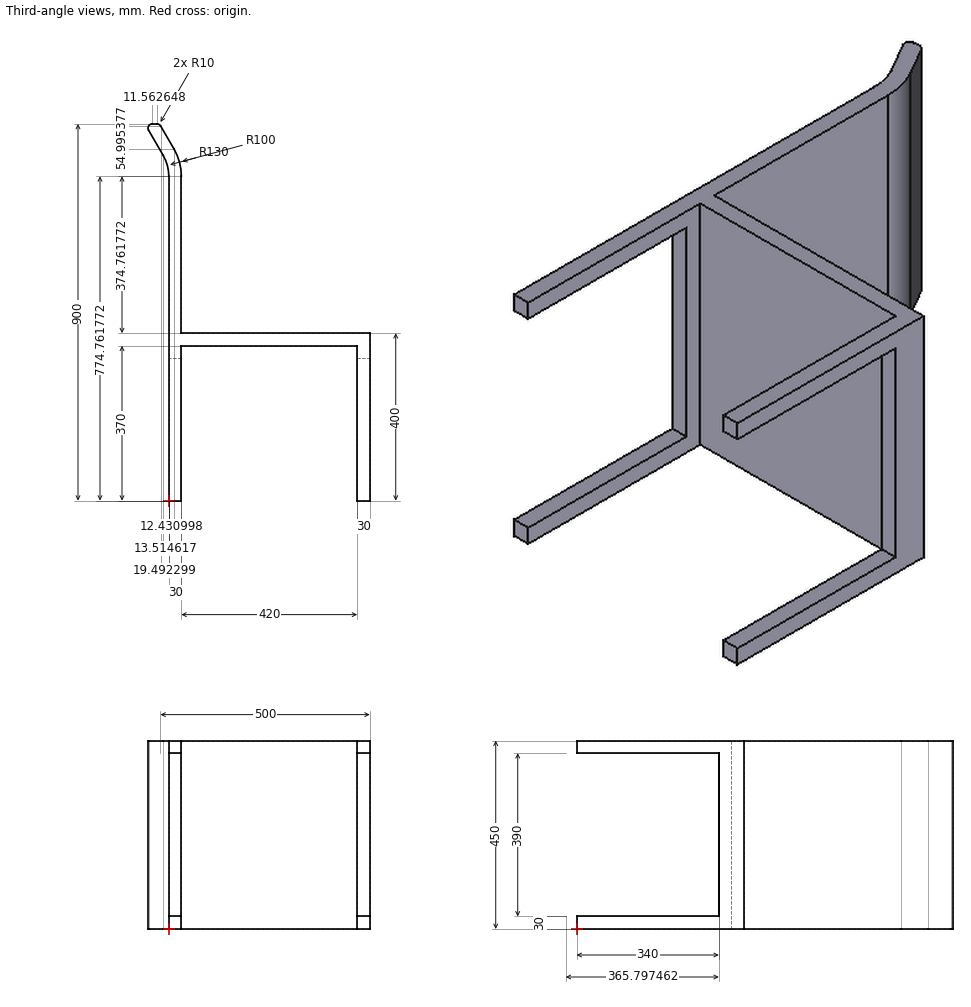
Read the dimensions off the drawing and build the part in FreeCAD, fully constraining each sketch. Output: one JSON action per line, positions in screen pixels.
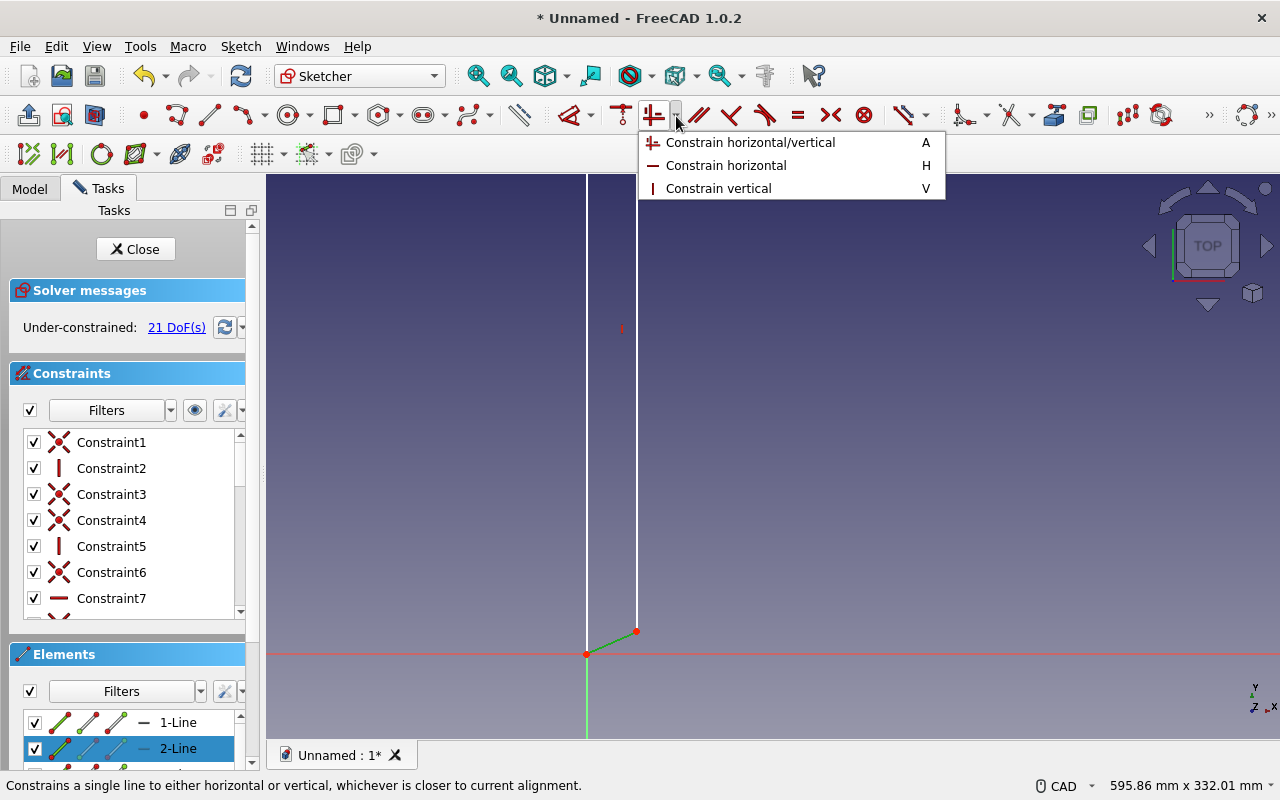
{"action": "left_click", "coordinate": [792, 166]}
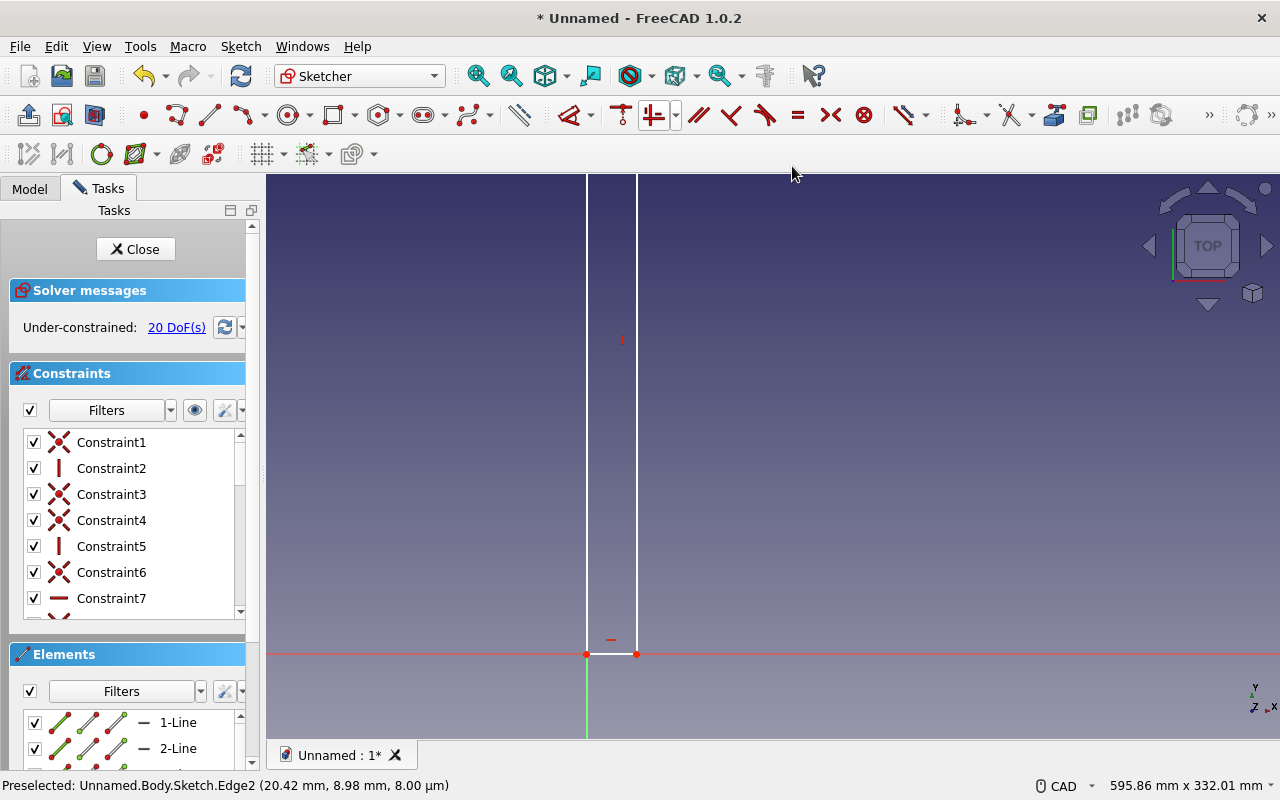
{"action": "scroll", "coordinate": [623, 642], "scroll_direction": "down", "scroll_amount": 7}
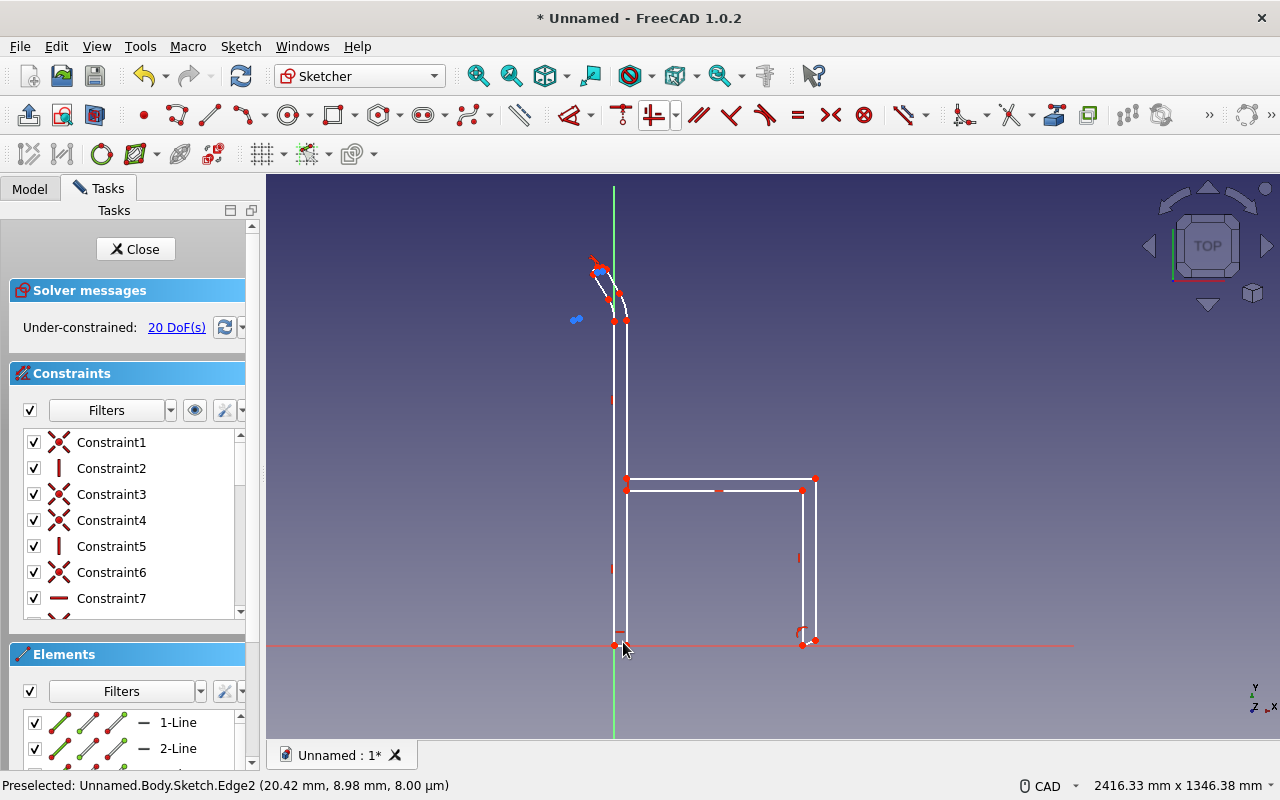
{"action": "scroll", "coordinate": [812, 642], "scroll_direction": "up", "scroll_amount": 7}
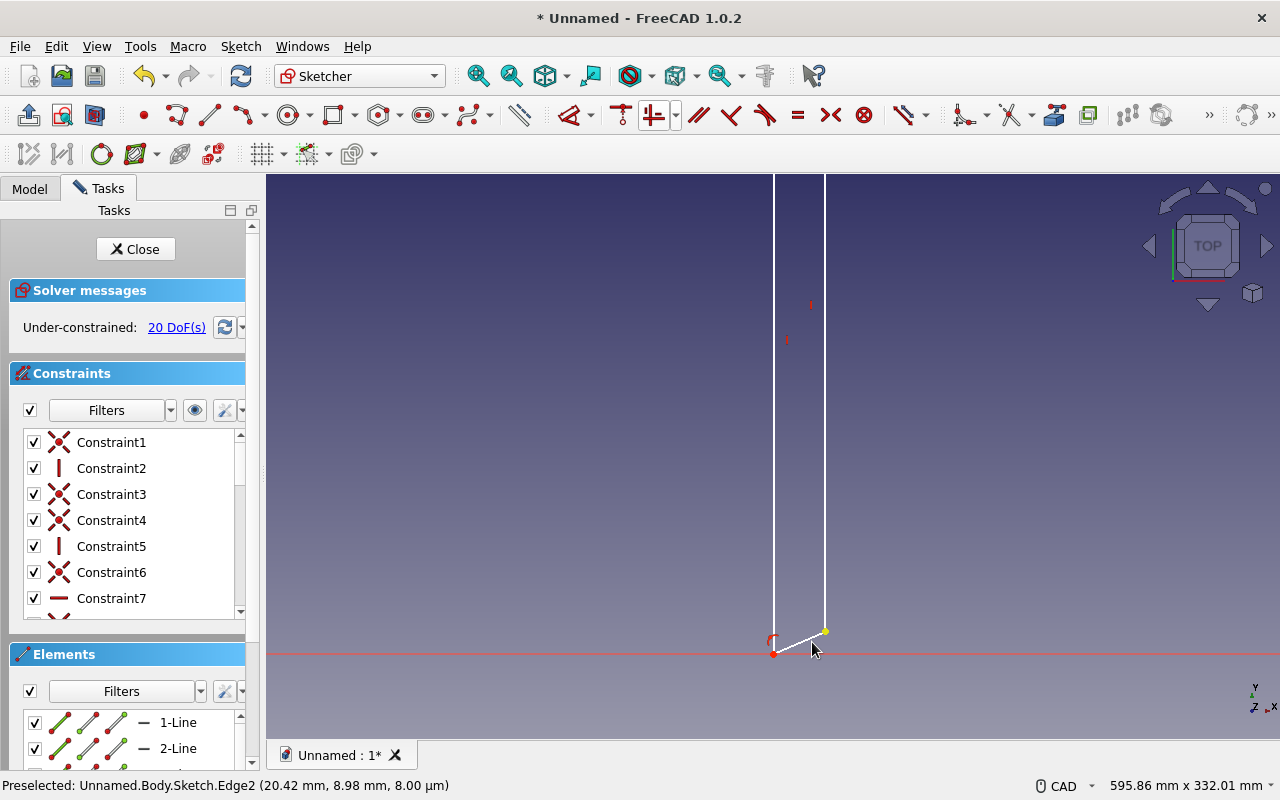
{"action": "left_click", "coordinate": [810, 639]}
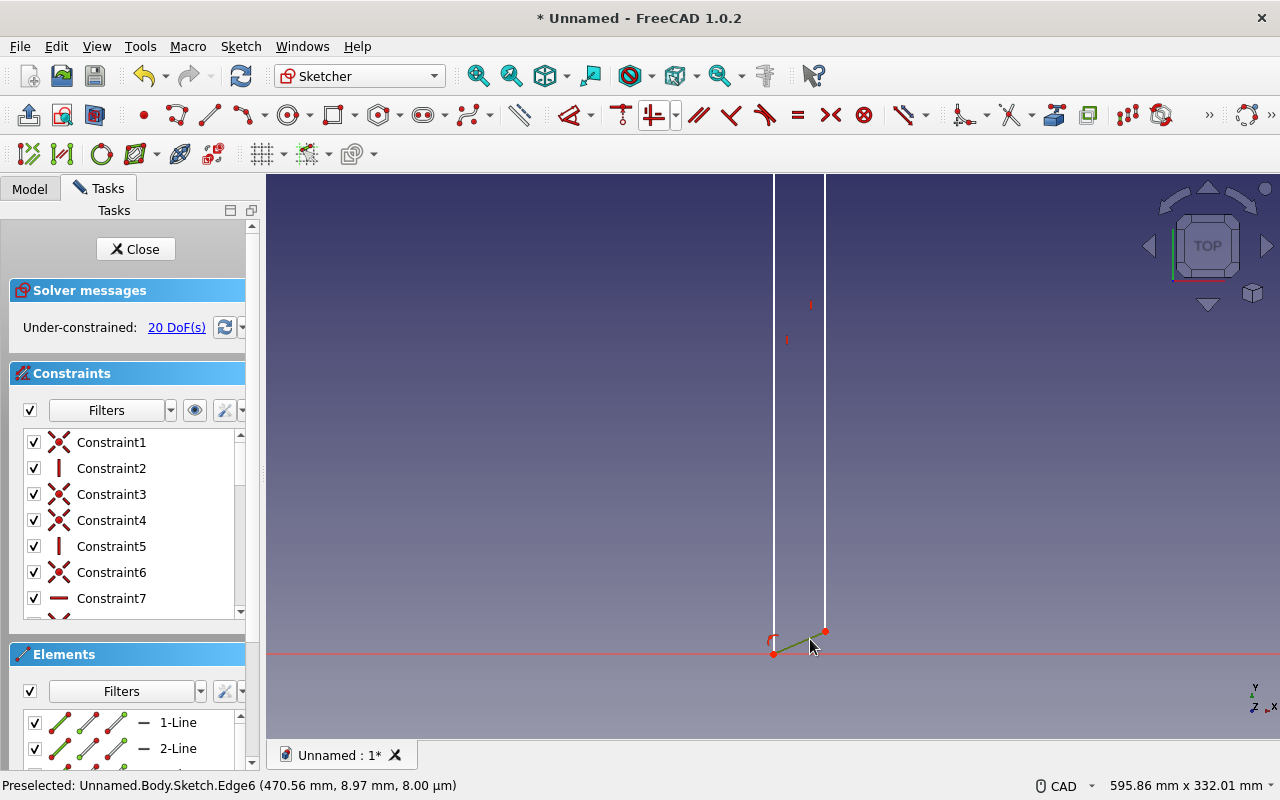
{"action": "left_click", "coordinate": [676, 116]}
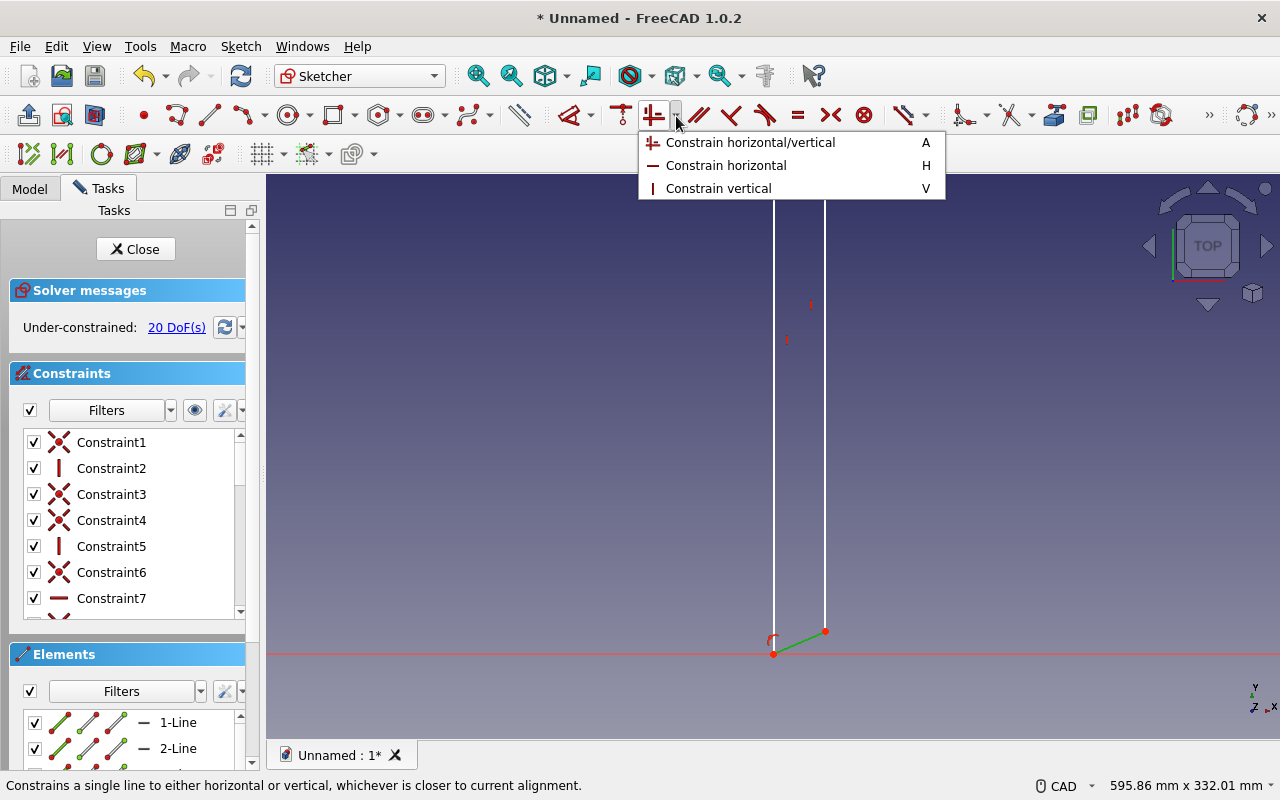
{"action": "left_click", "coordinate": [792, 166]}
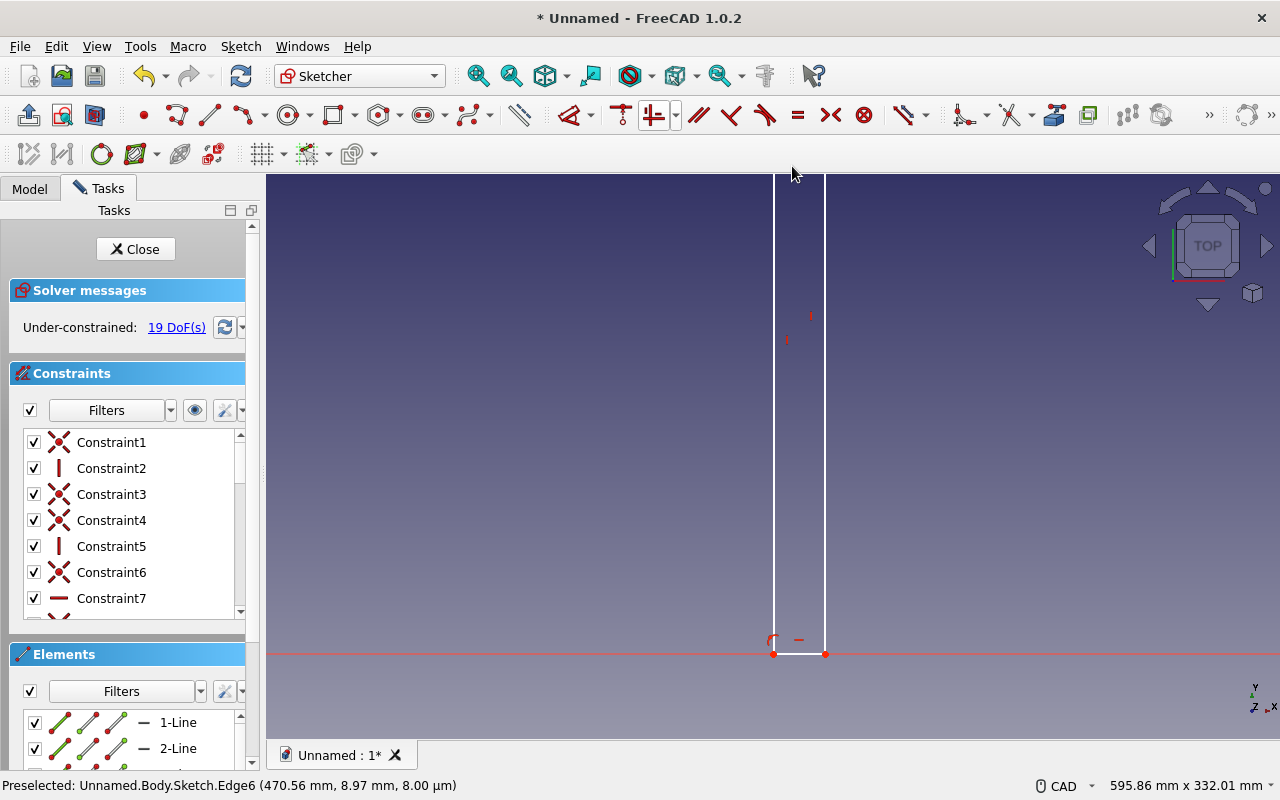
{"action": "scroll", "coordinate": [812, 642], "scroll_direction": "down", "scroll_amount": 7}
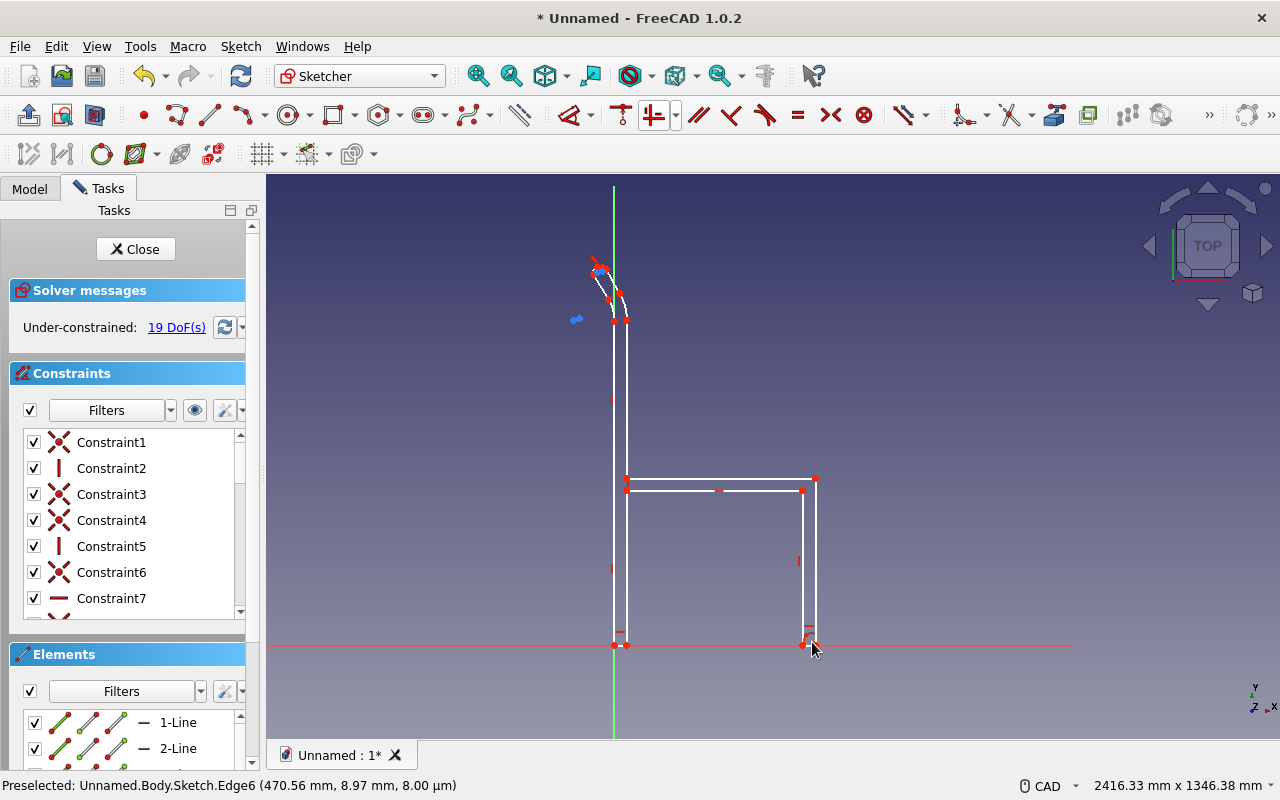
{"action": "scroll", "coordinate": [626, 312], "scroll_direction": "up", "scroll_amount": 3}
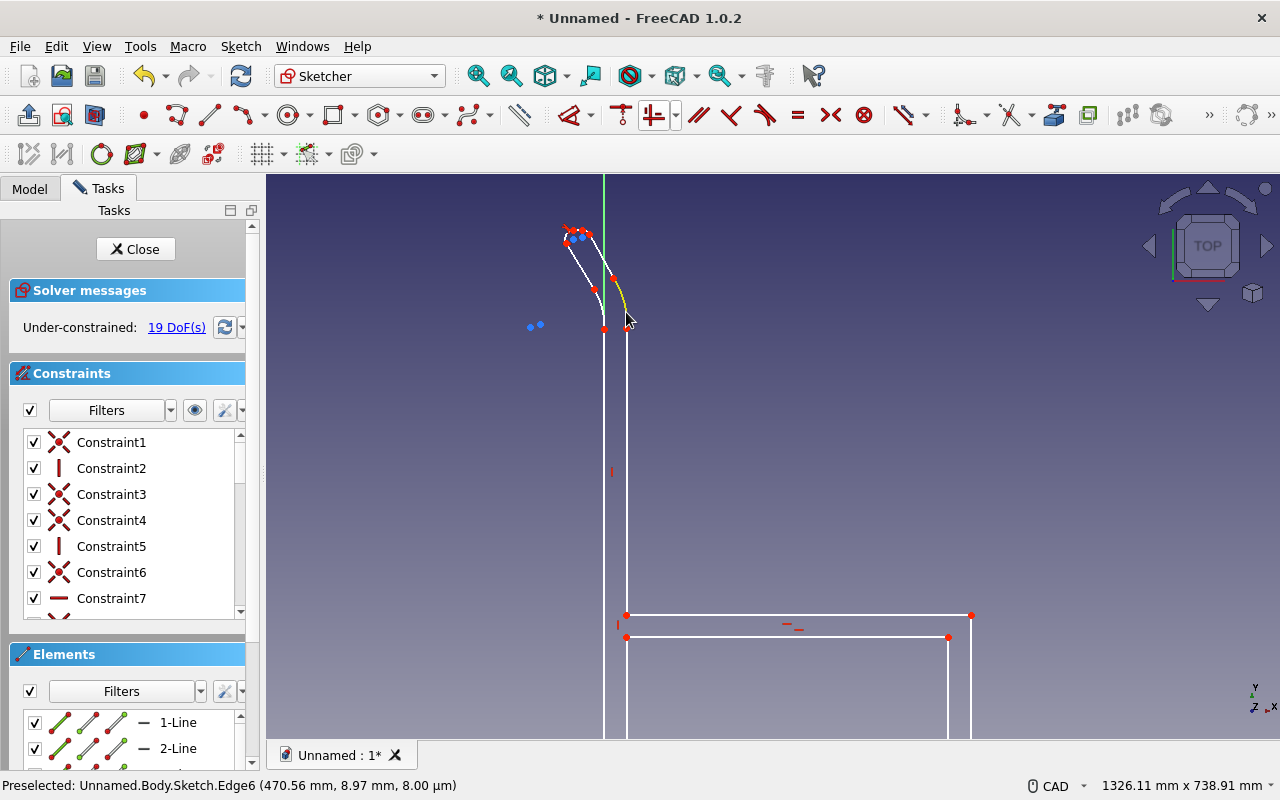
{"action": "left_click", "coordinate": [626, 312]}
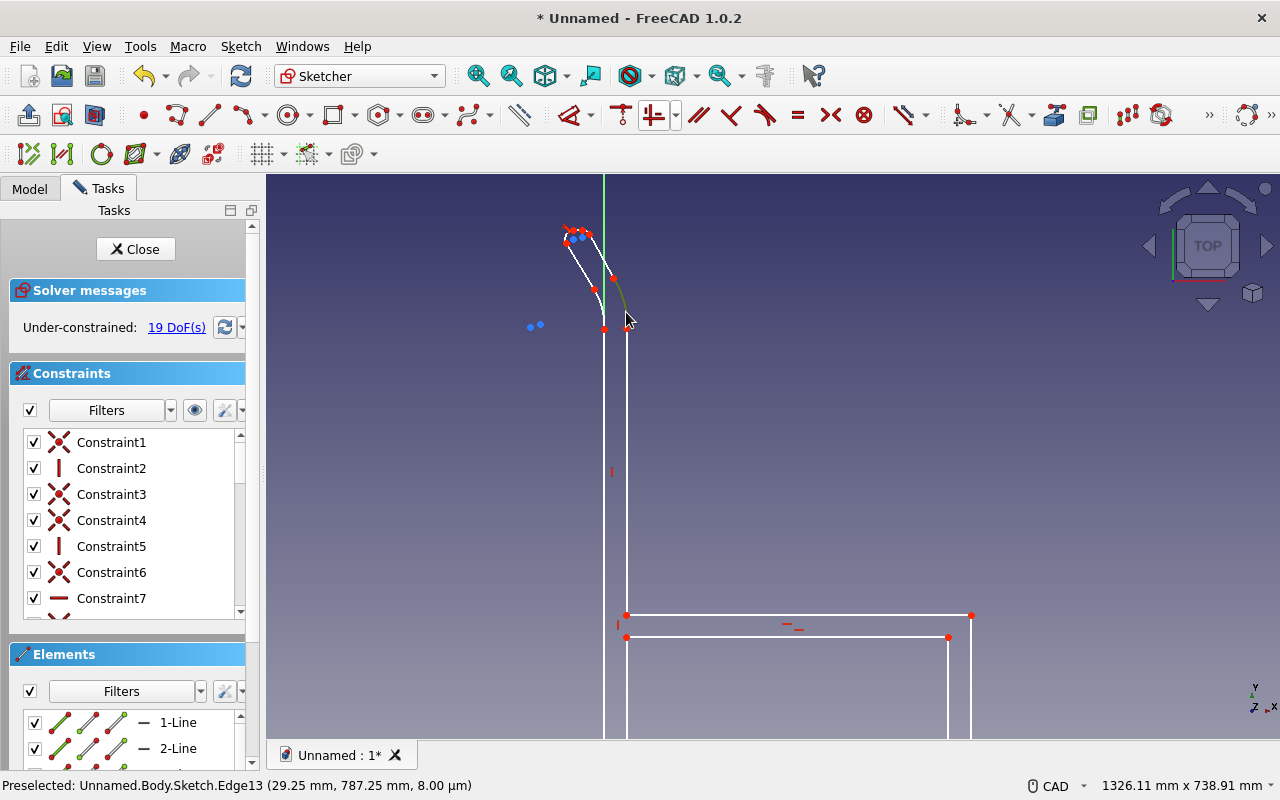
{"action": "left_click", "coordinate": [604, 317]}